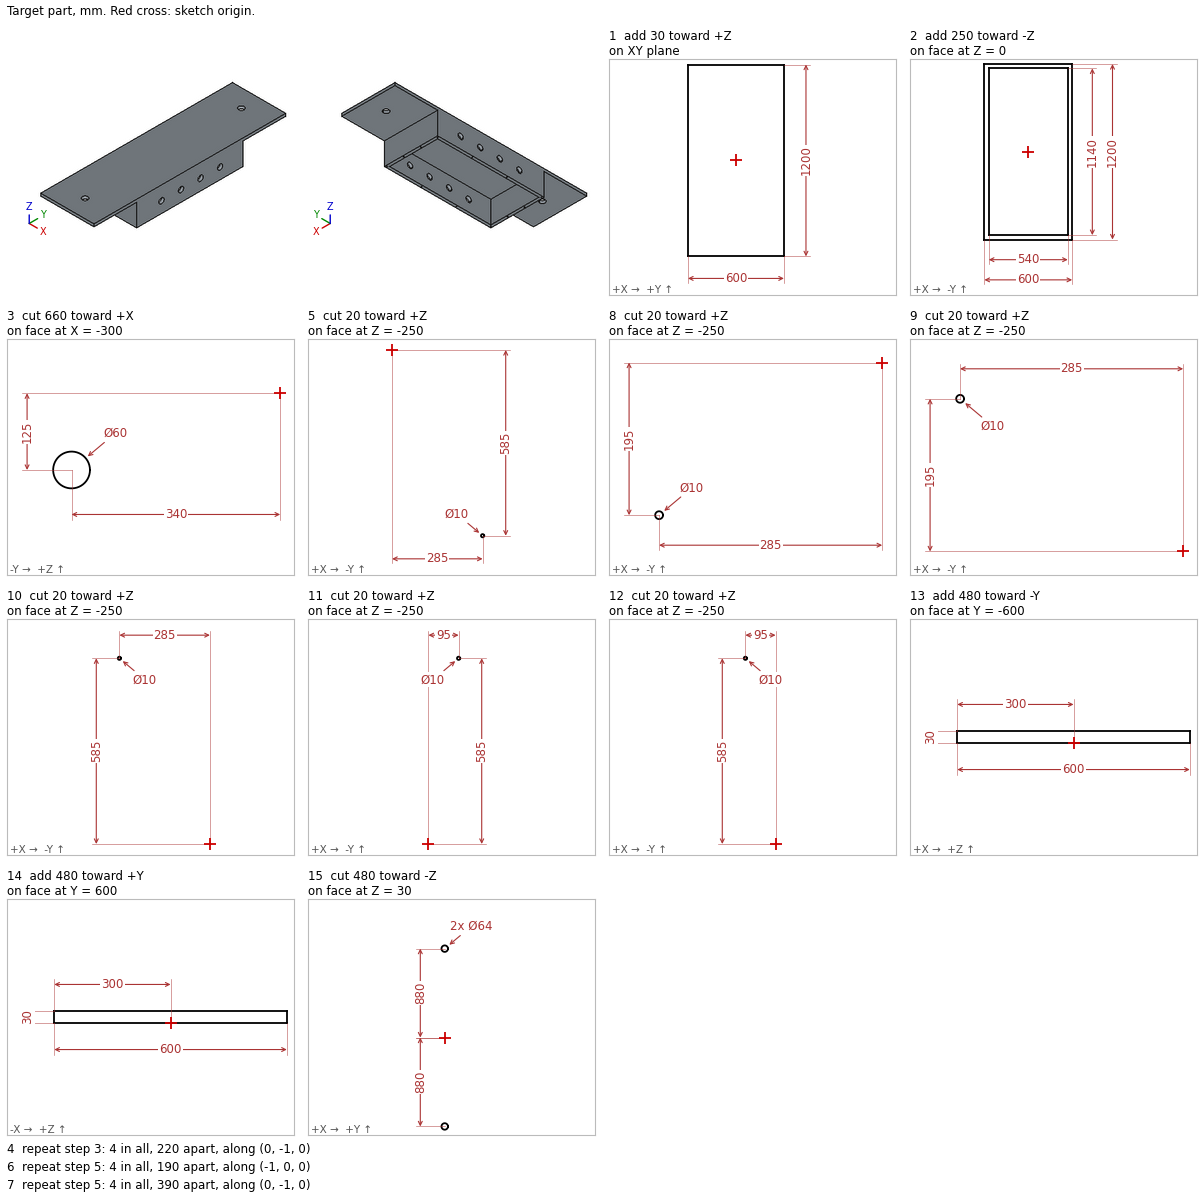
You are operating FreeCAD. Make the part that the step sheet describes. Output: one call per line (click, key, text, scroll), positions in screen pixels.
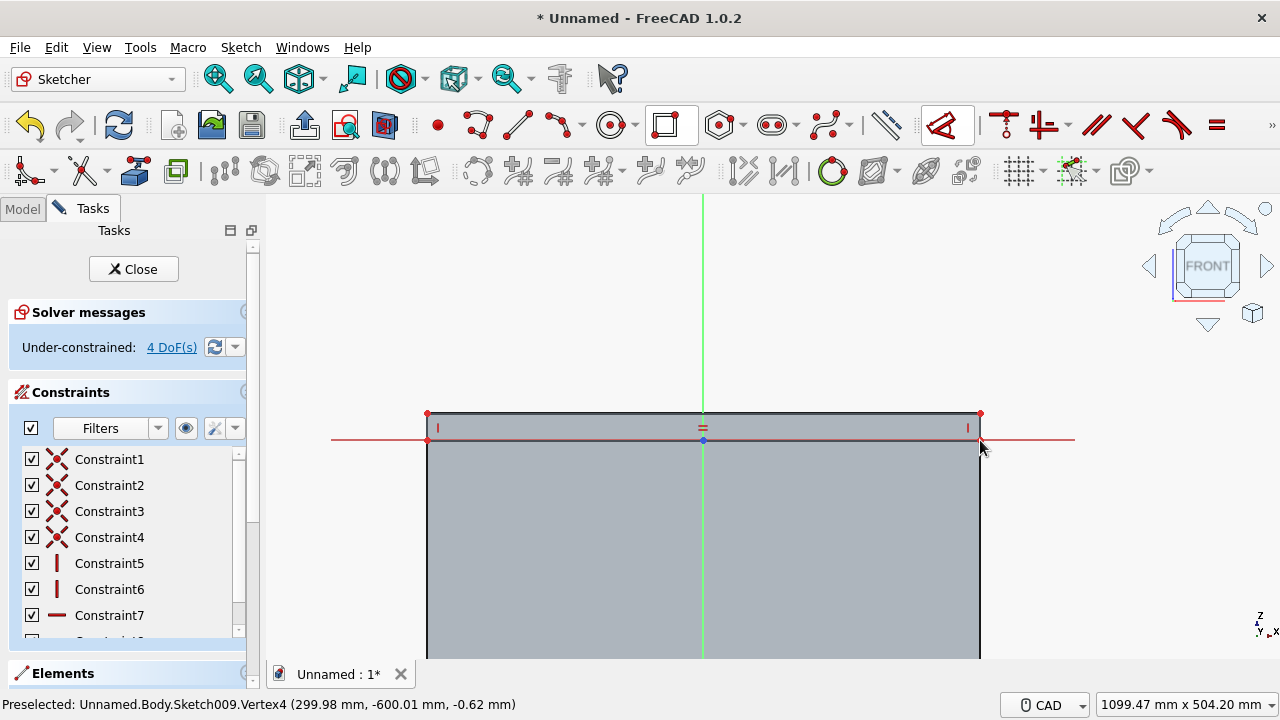
click(427, 441)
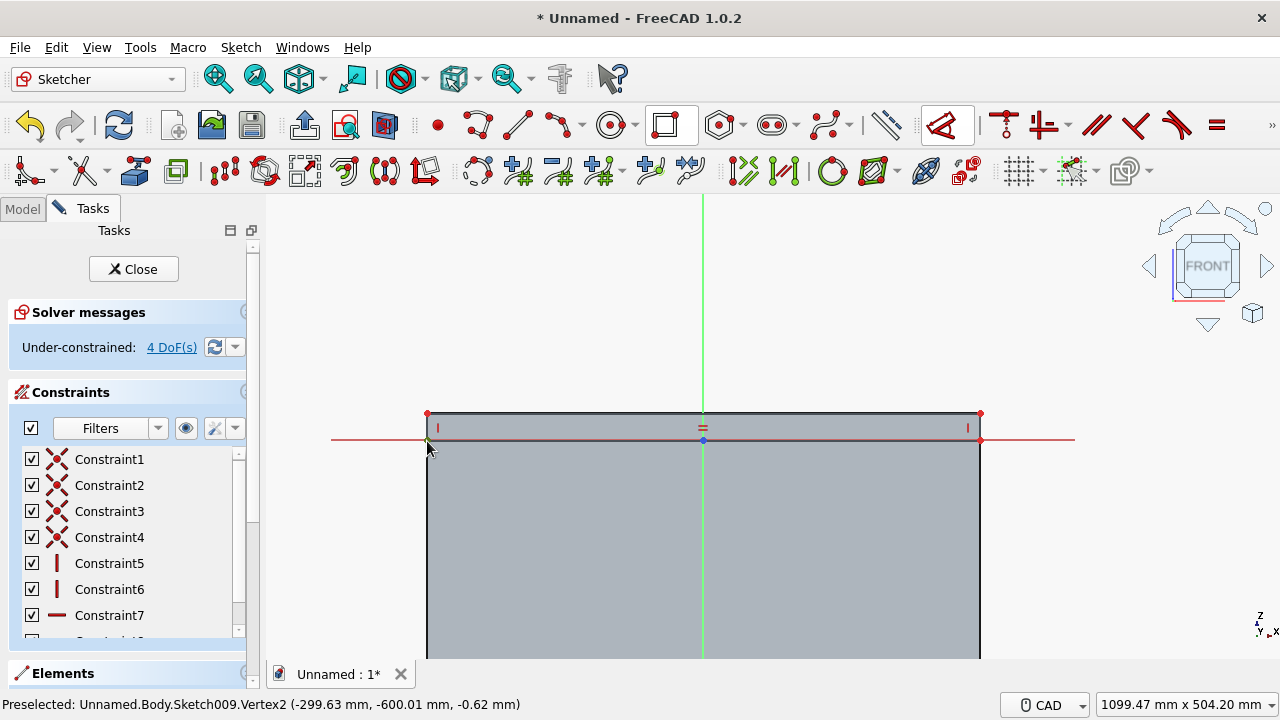
click(353, 440)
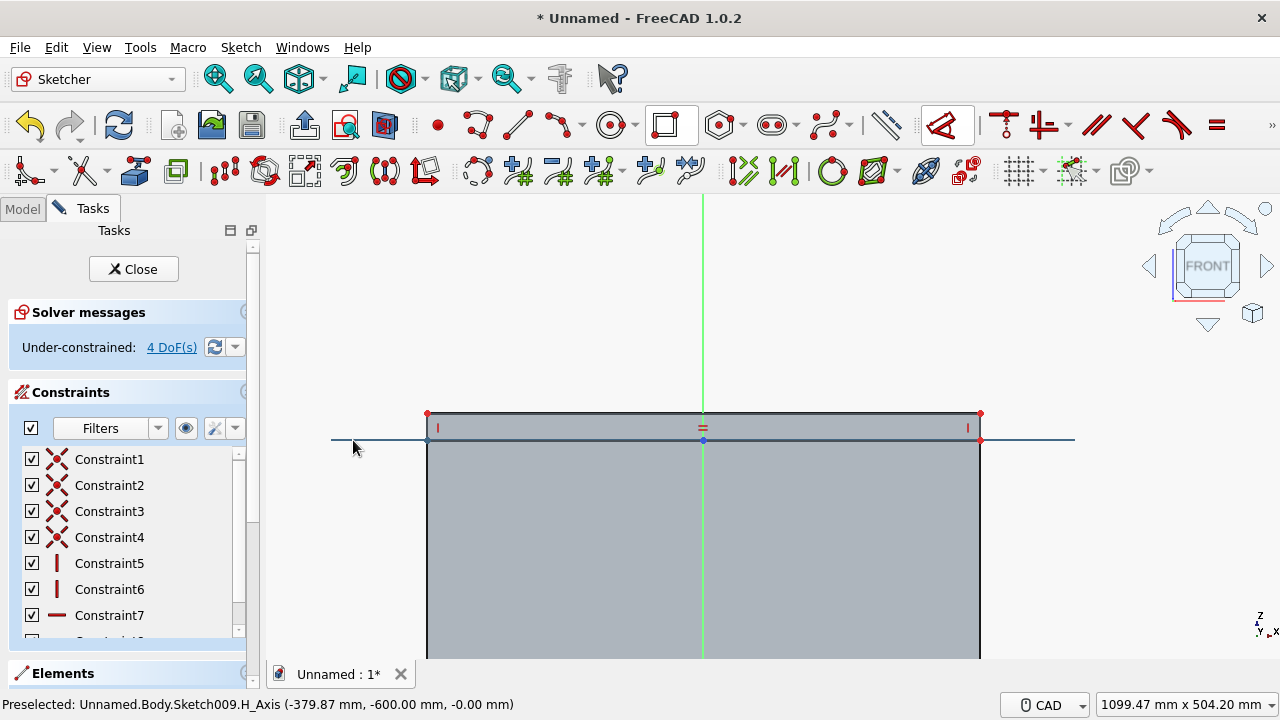
click(1004, 126)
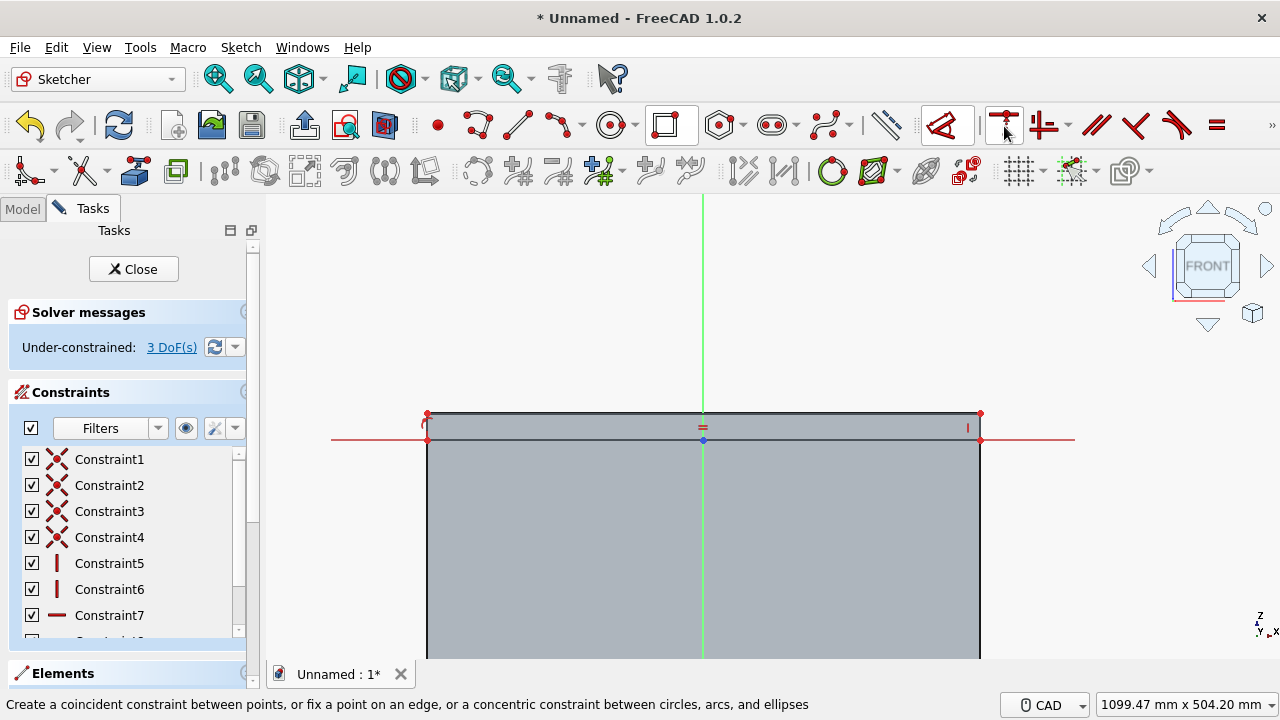
scroll(427, 425, up, 2)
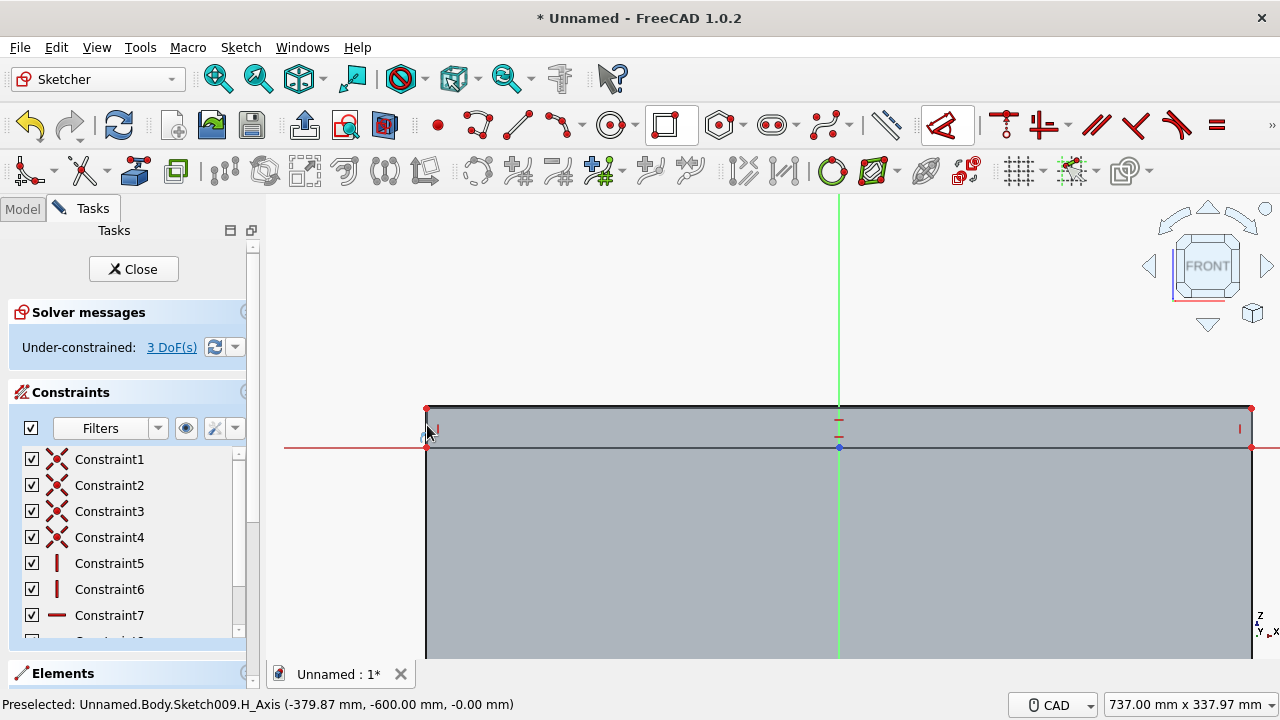
click(427, 424)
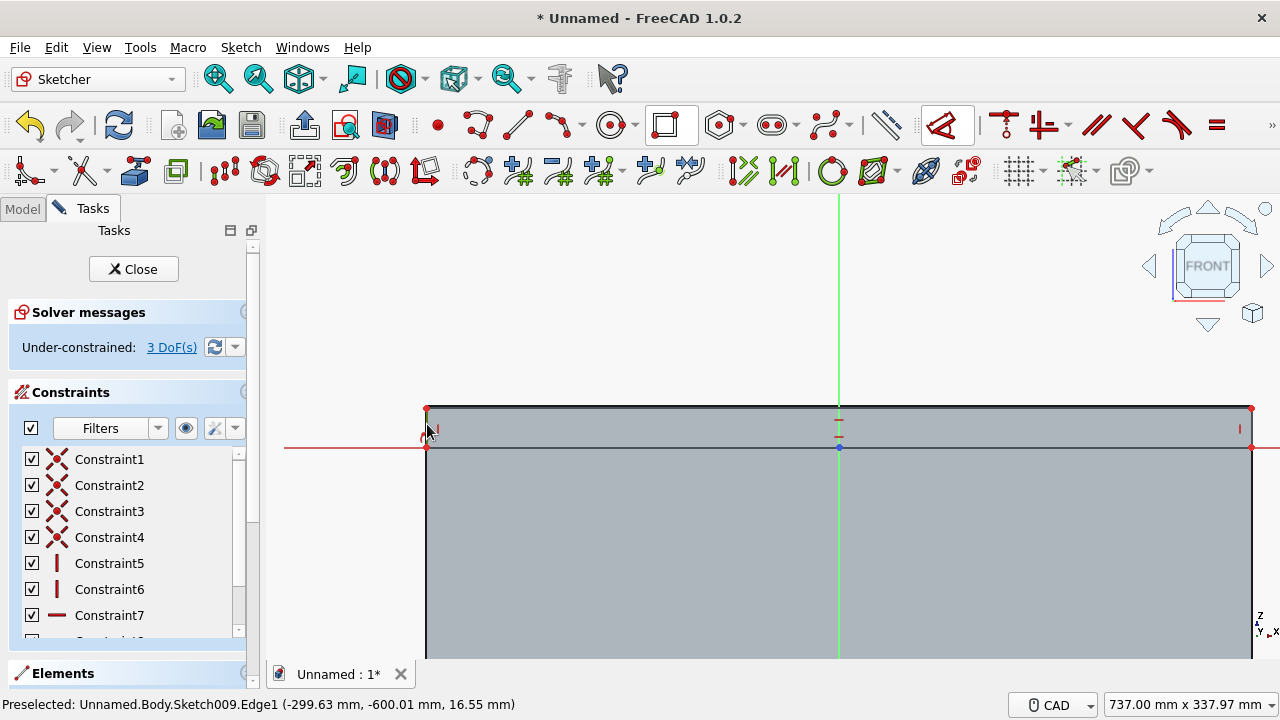
click(968, 126)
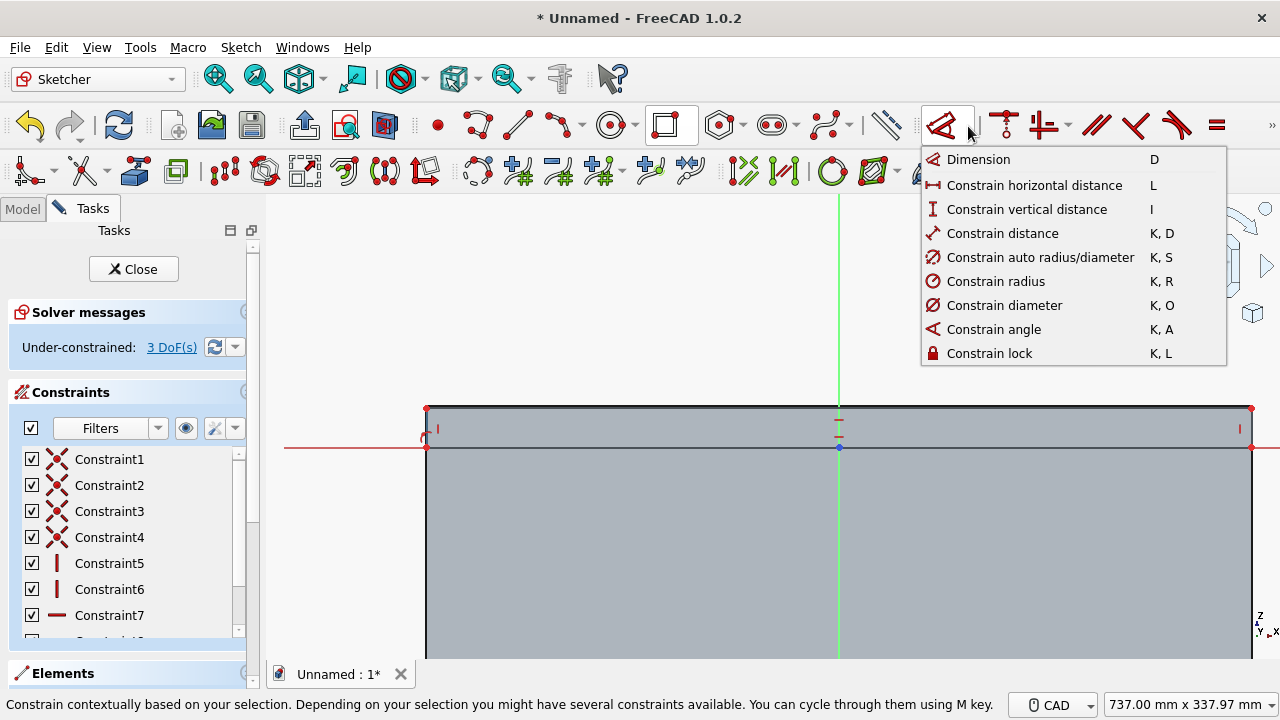
click(1074, 209)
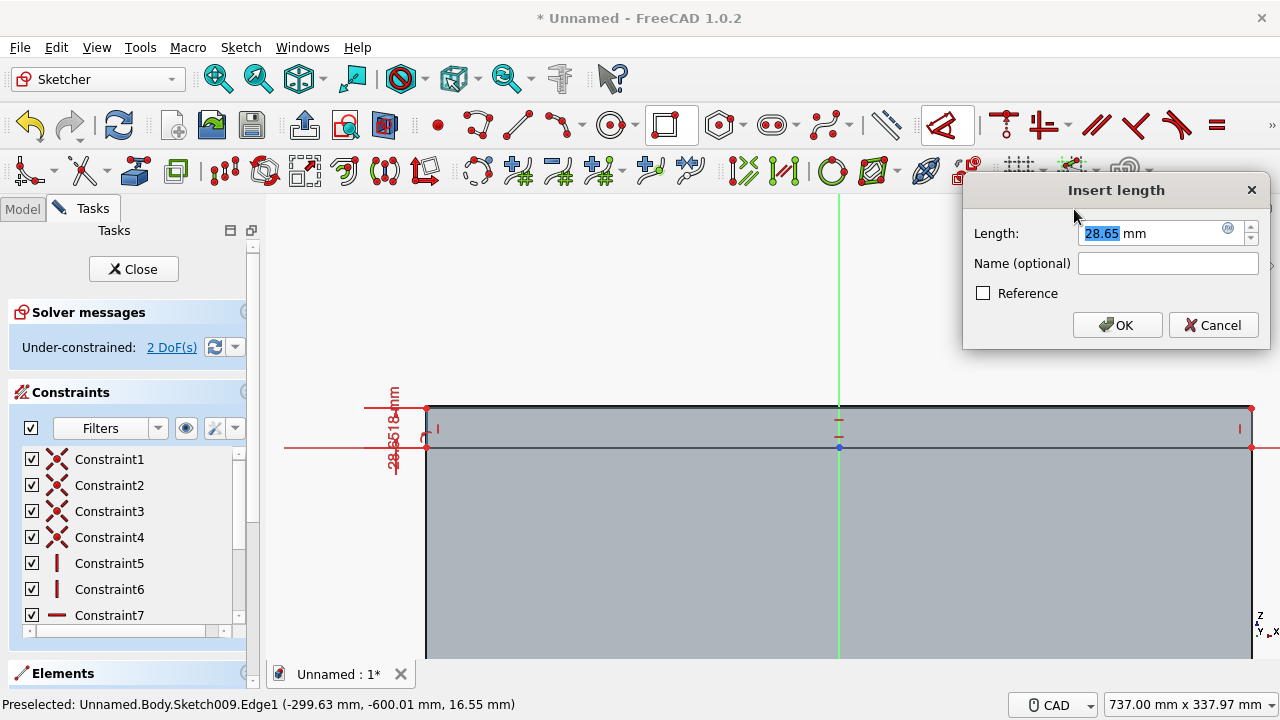
text(30)
key(Return)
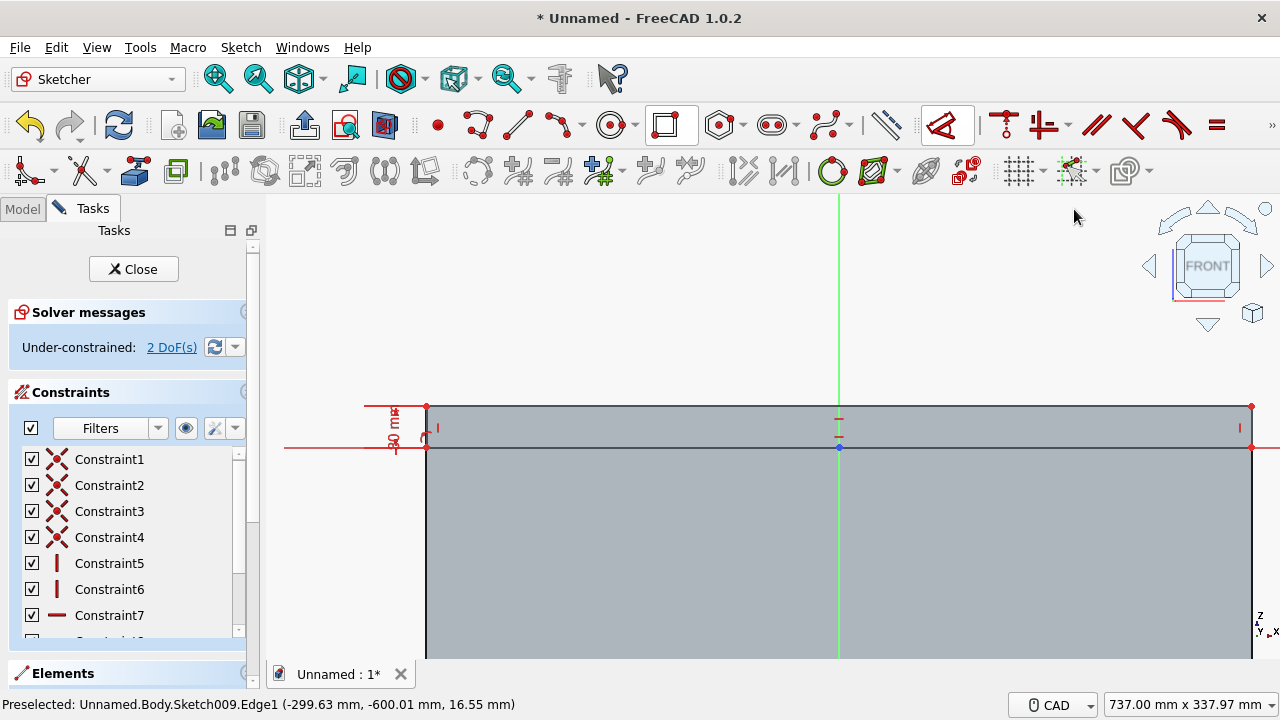
click(674, 448)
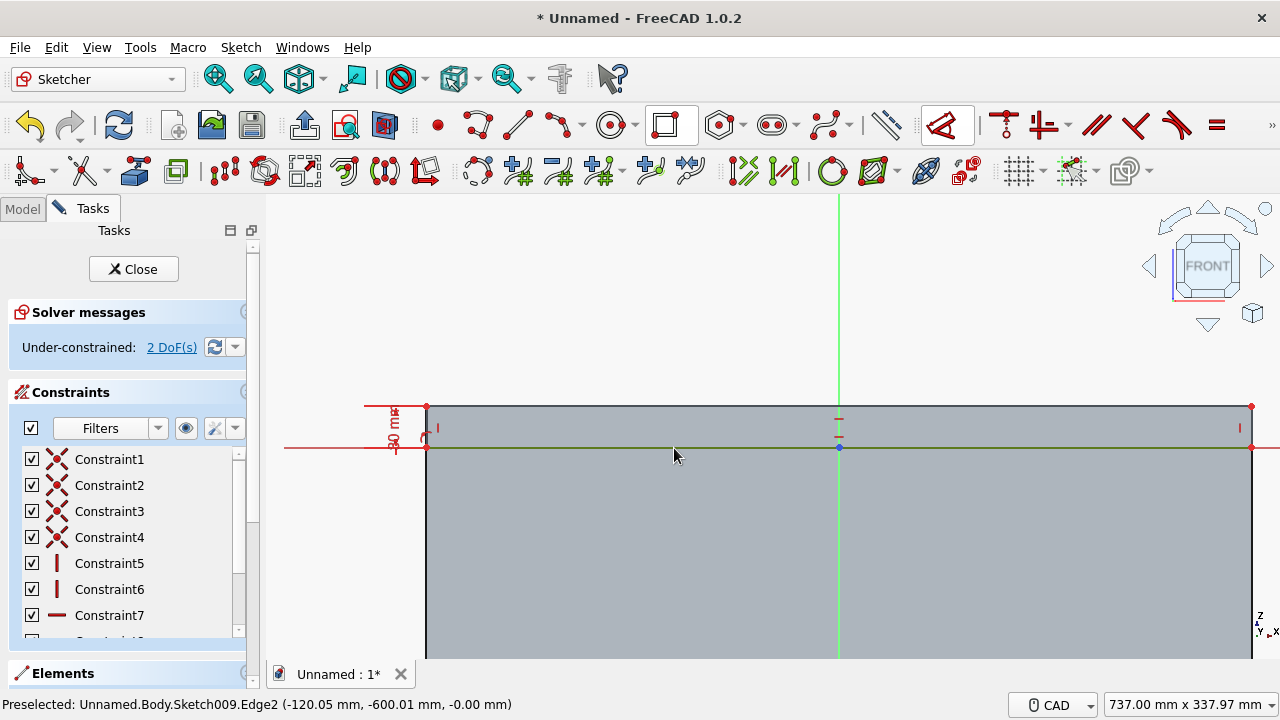
click(968, 126)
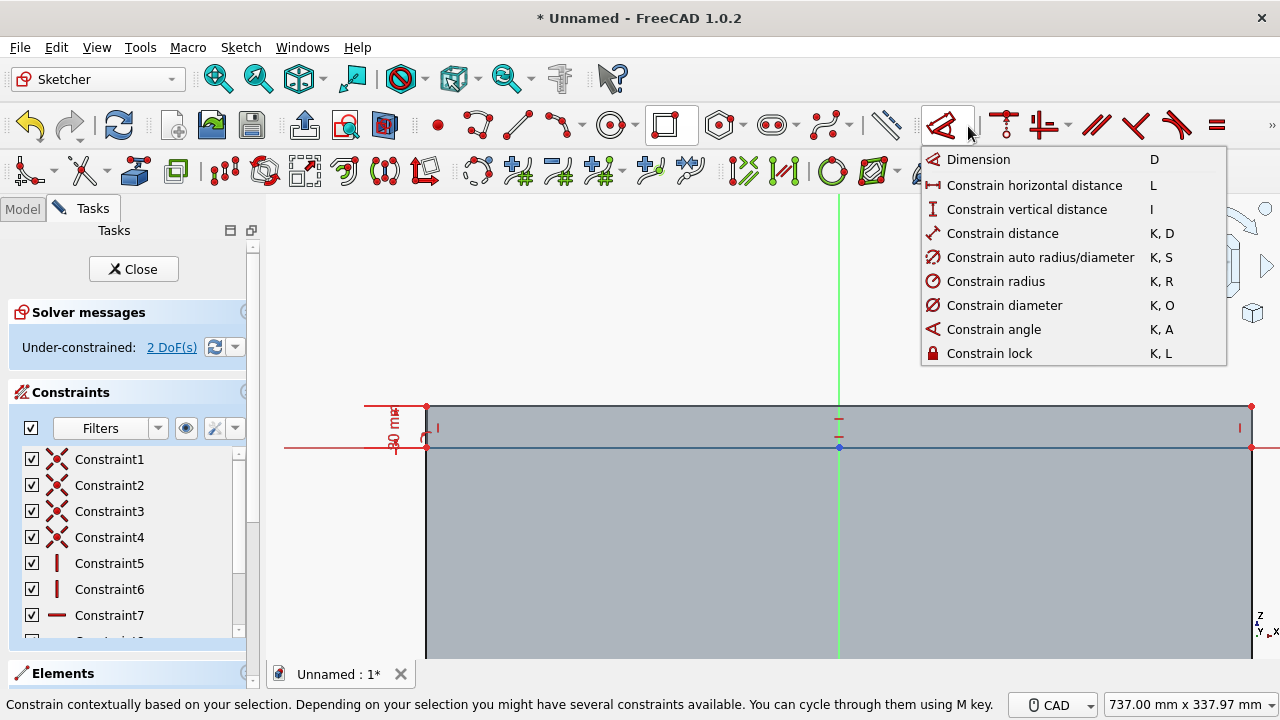
click(1074, 185)